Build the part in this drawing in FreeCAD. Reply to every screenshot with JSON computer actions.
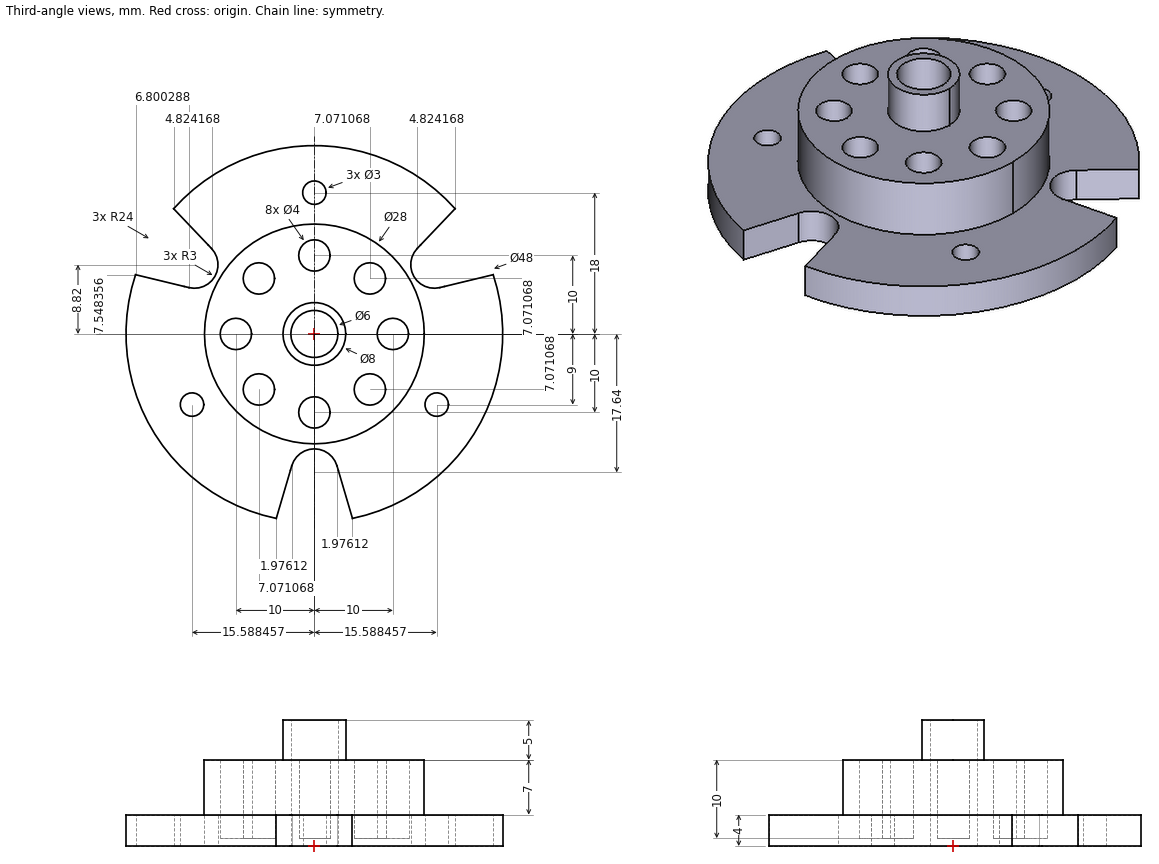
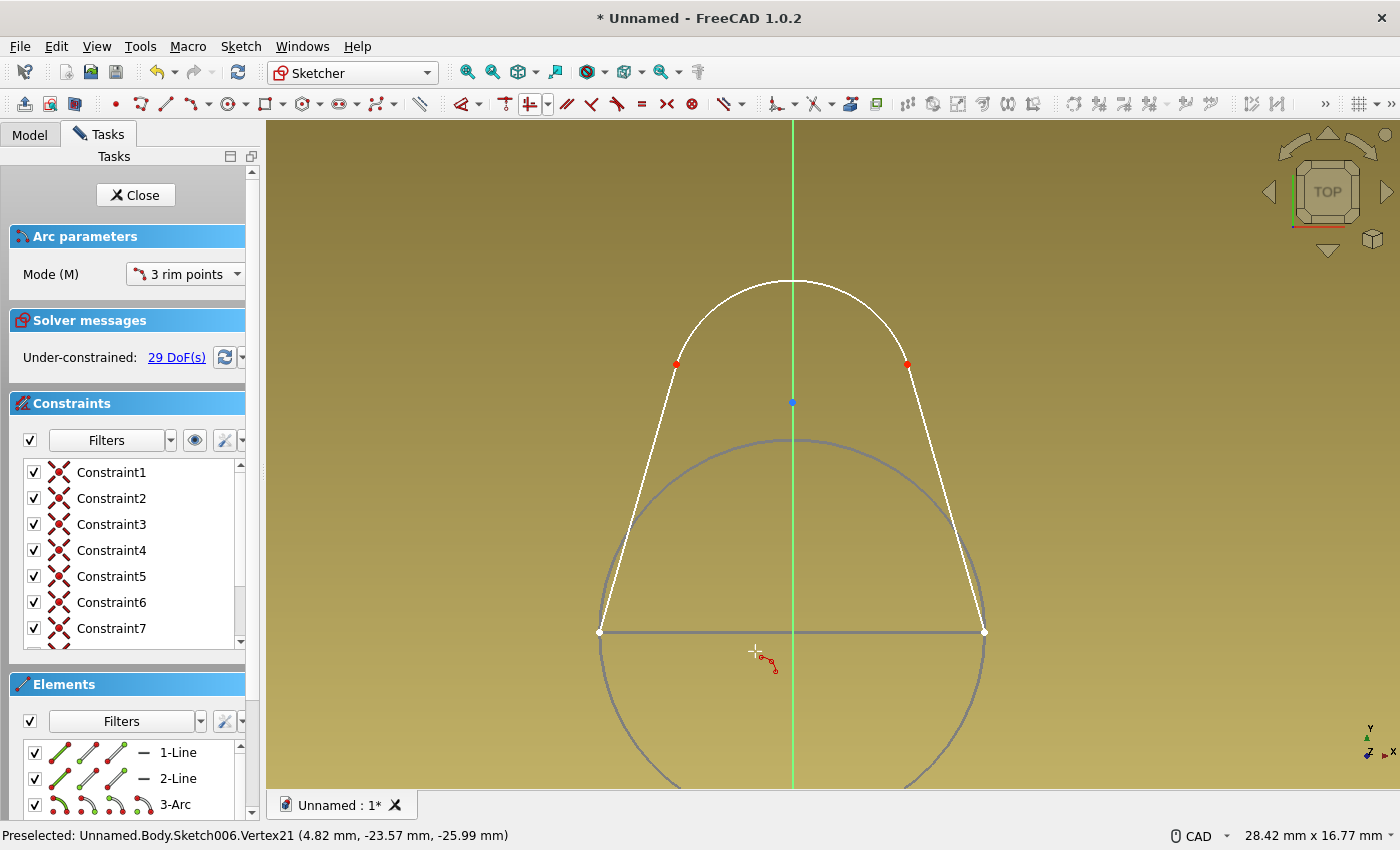
{"action": "left_click", "coordinate": [754, 649]}
{"action": "key", "text": "Escape"}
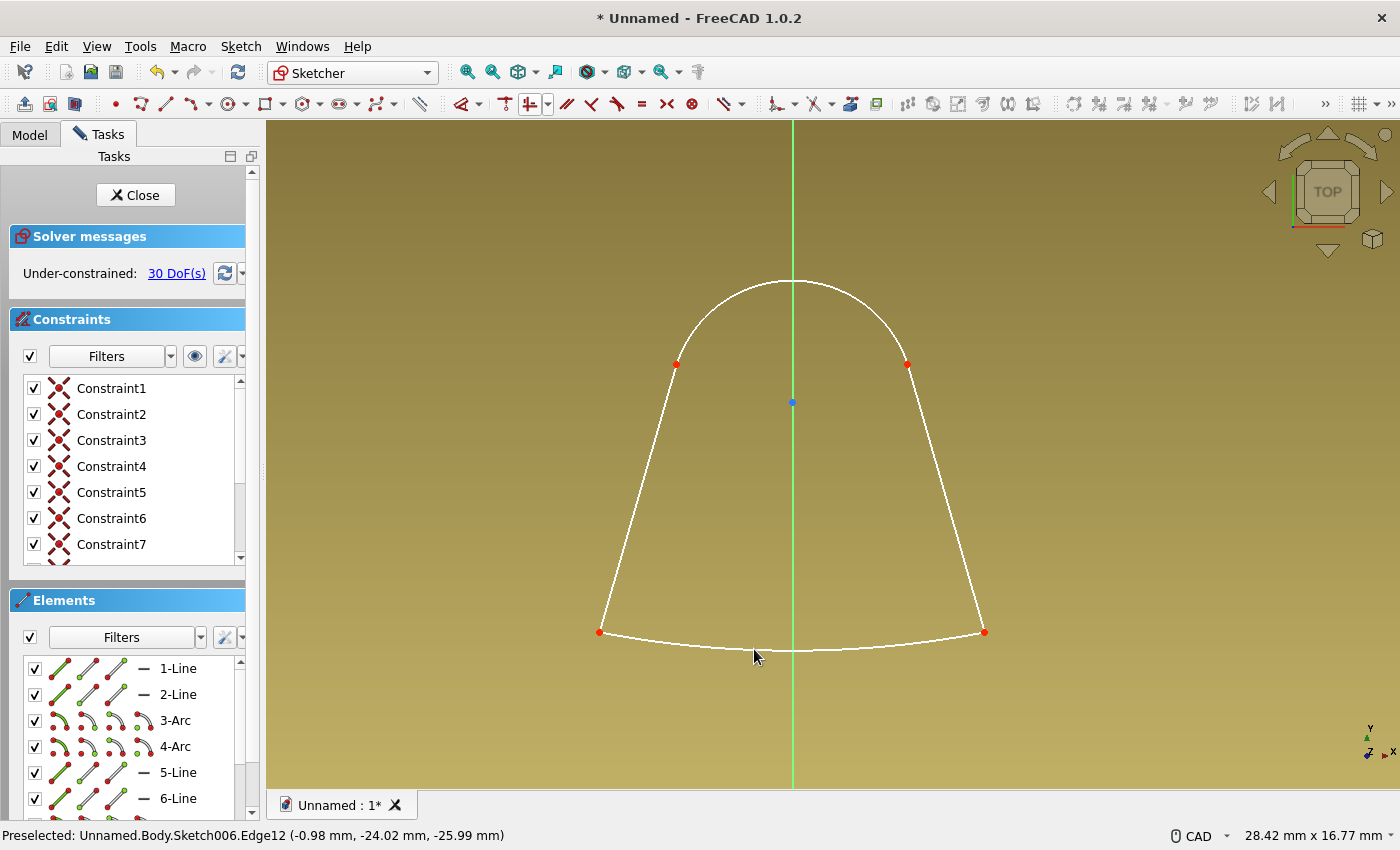
{"action": "scroll", "coordinate": [755, 652], "scroll_direction": "down", "scroll_amount": 7}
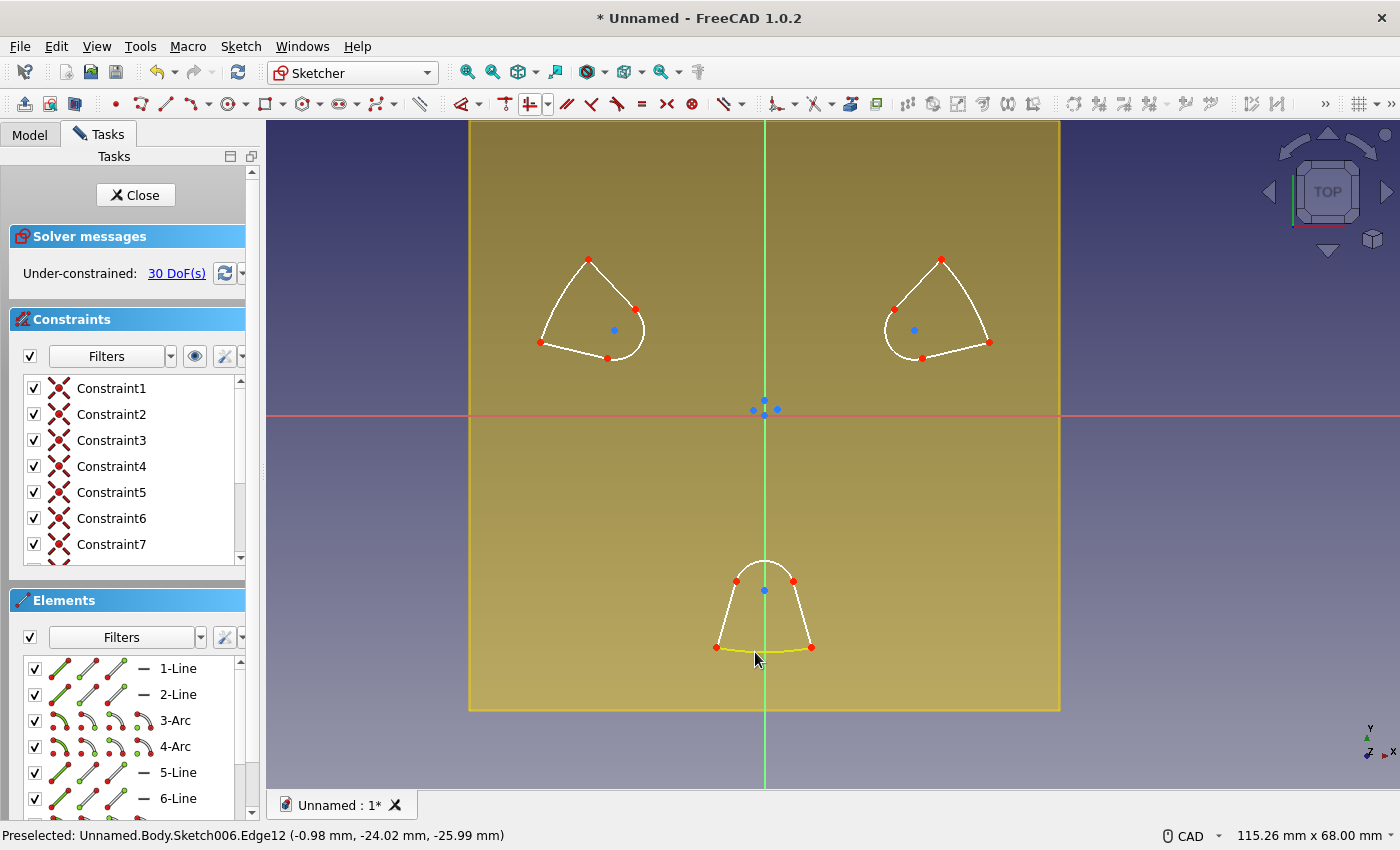
{"action": "left_click", "coordinate": [560, 348]}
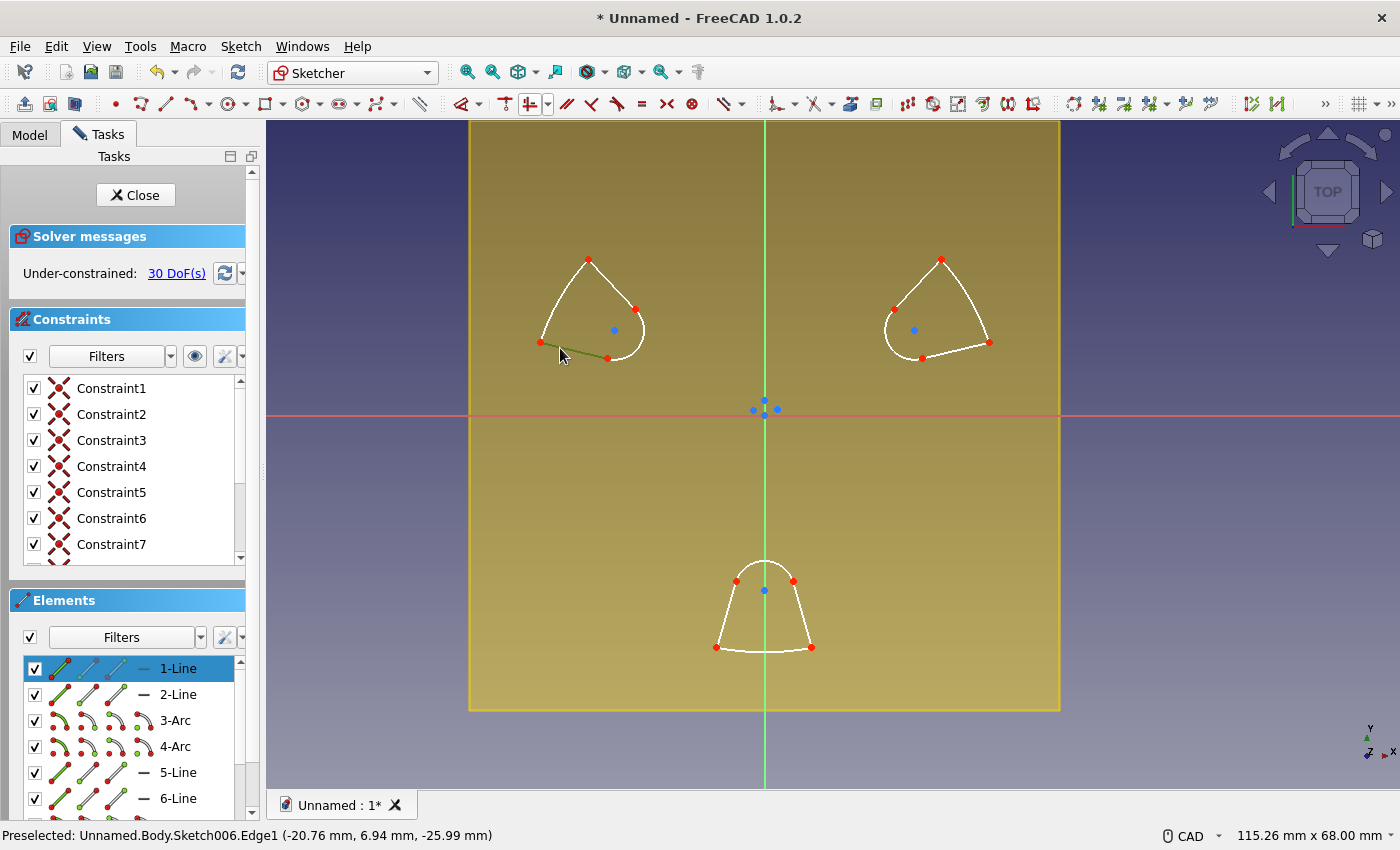
{"action": "left_click", "coordinate": [630, 356]}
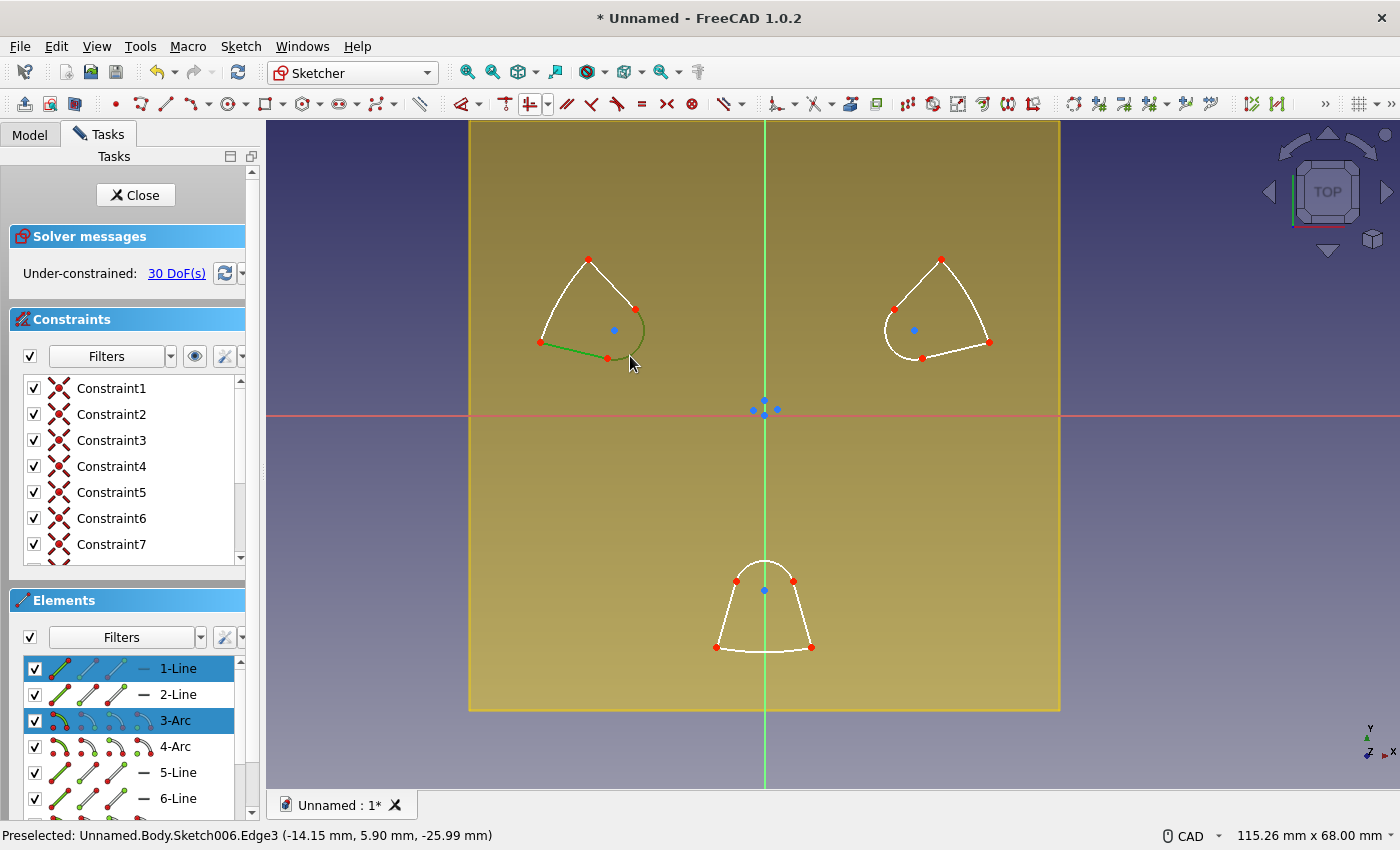
{"action": "key", "text": "t"}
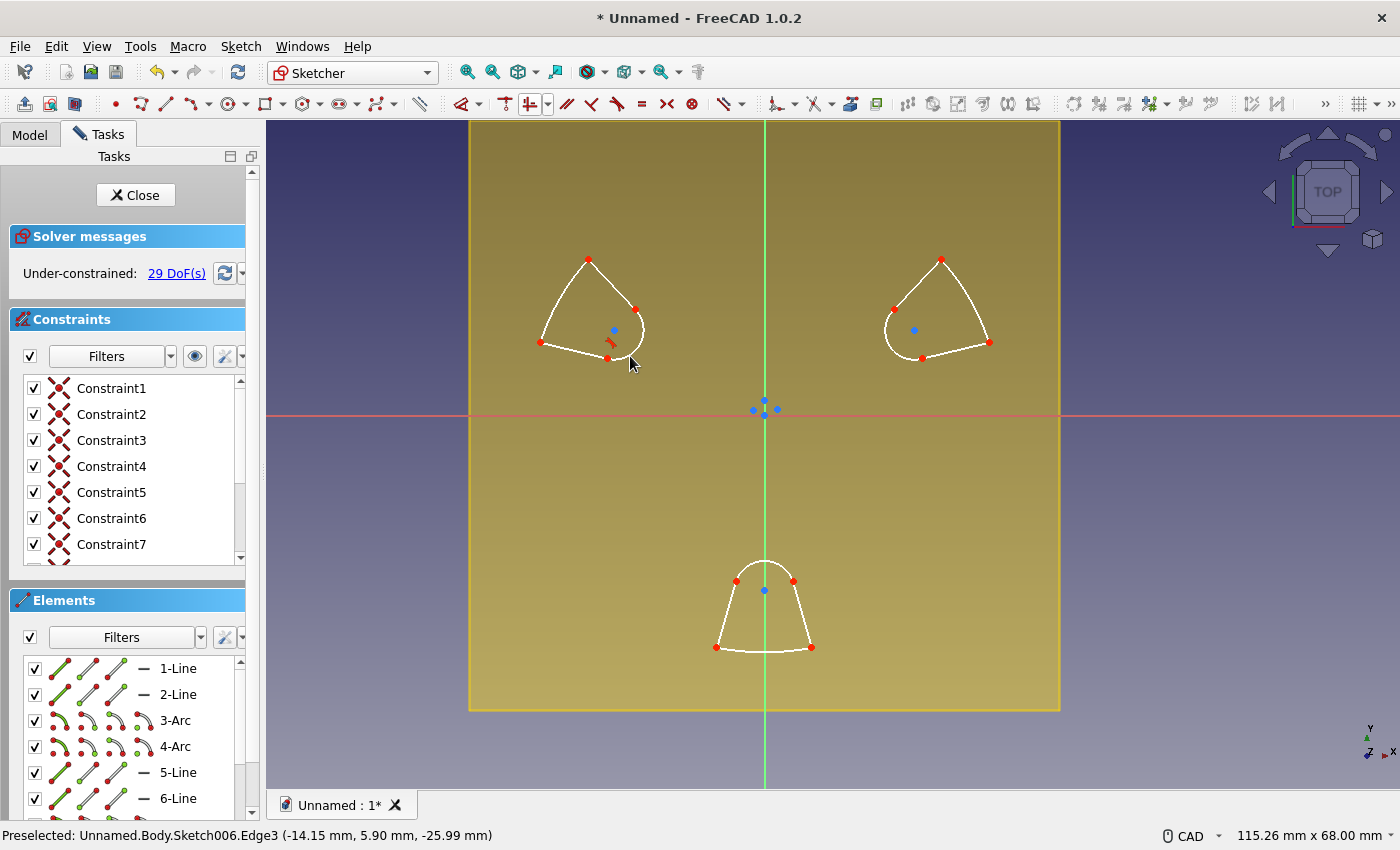
{"action": "left_click", "coordinate": [621, 295]}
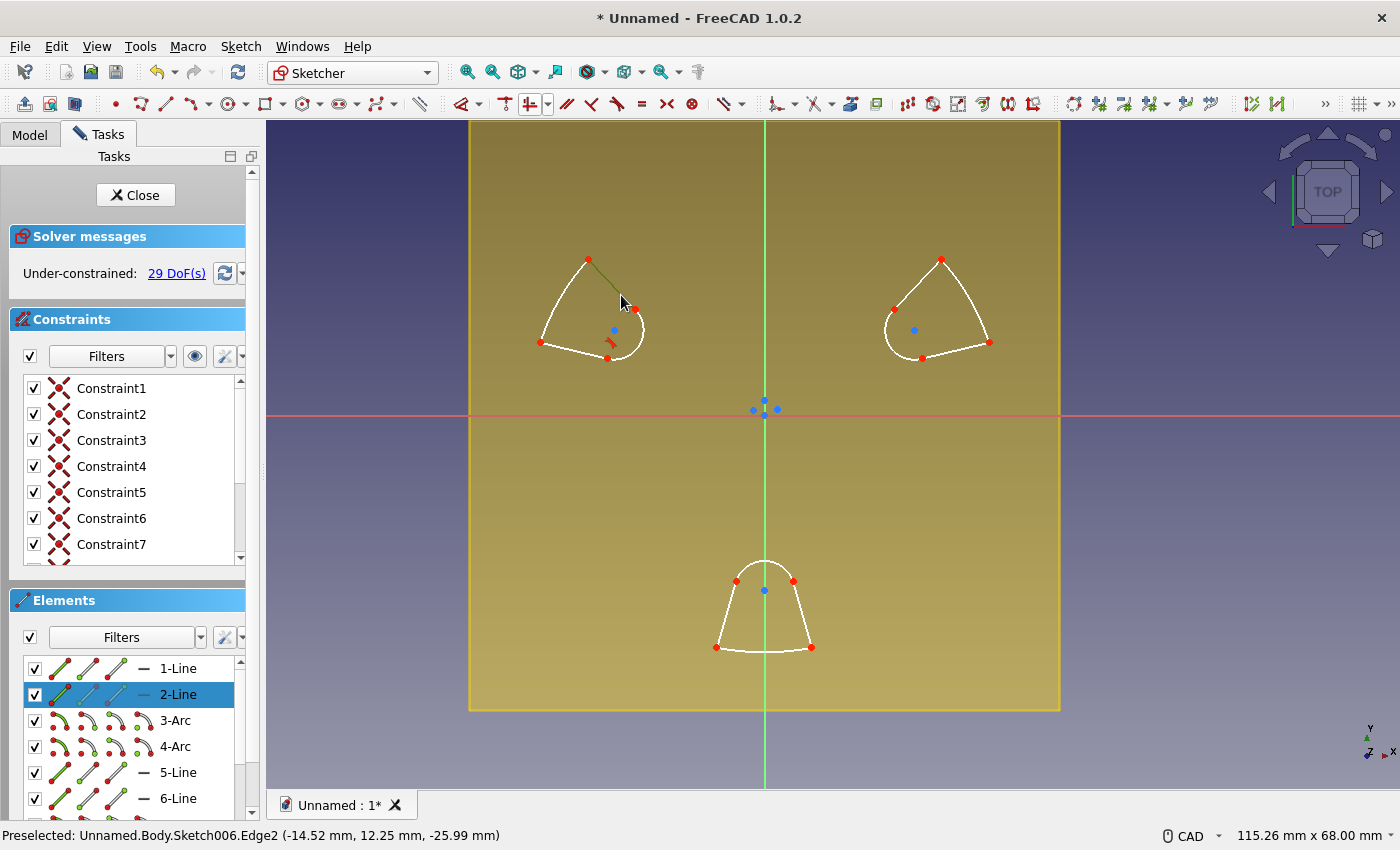
{"action": "left_click", "coordinate": [629, 355]}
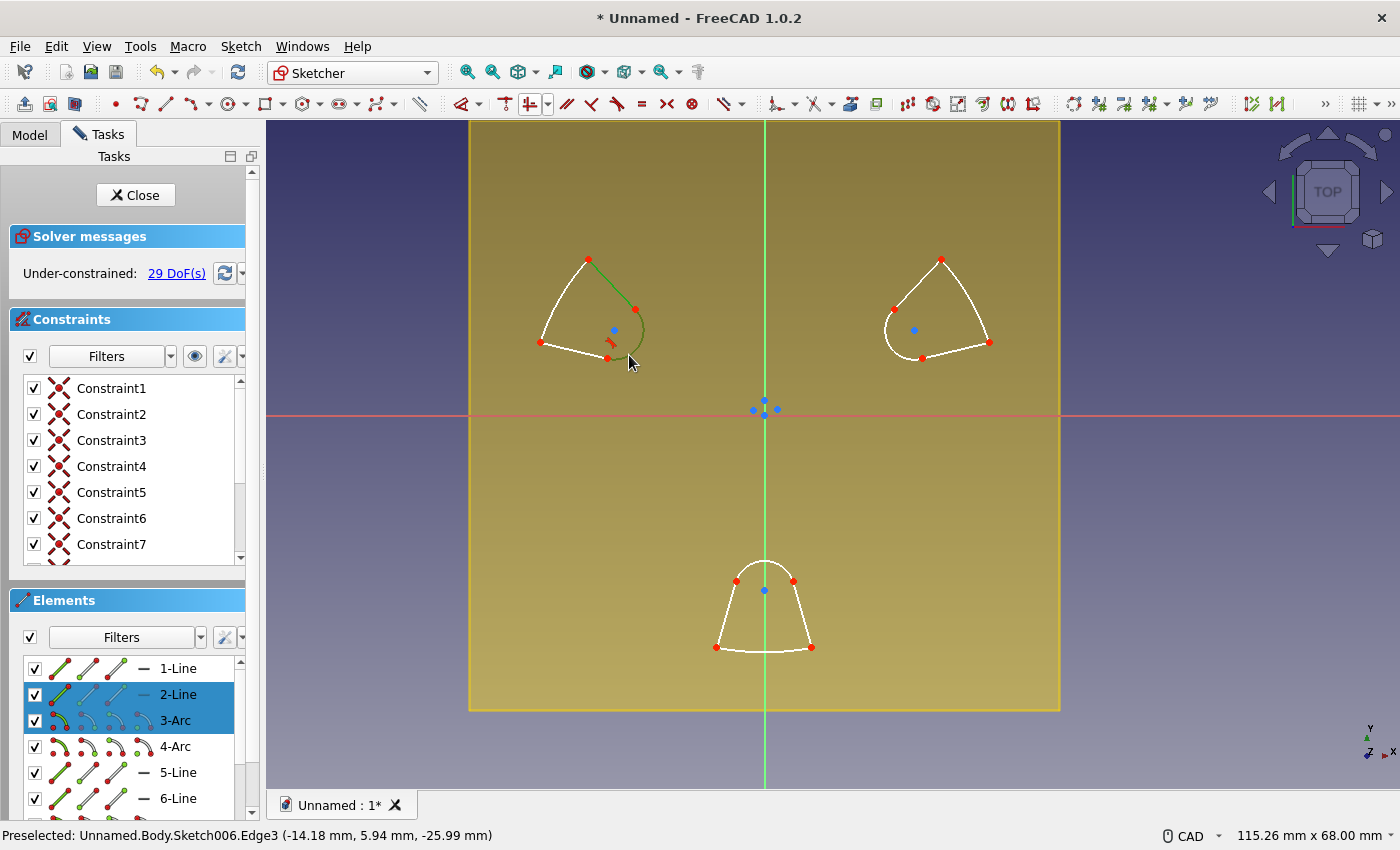
{"action": "key", "text": "t"}